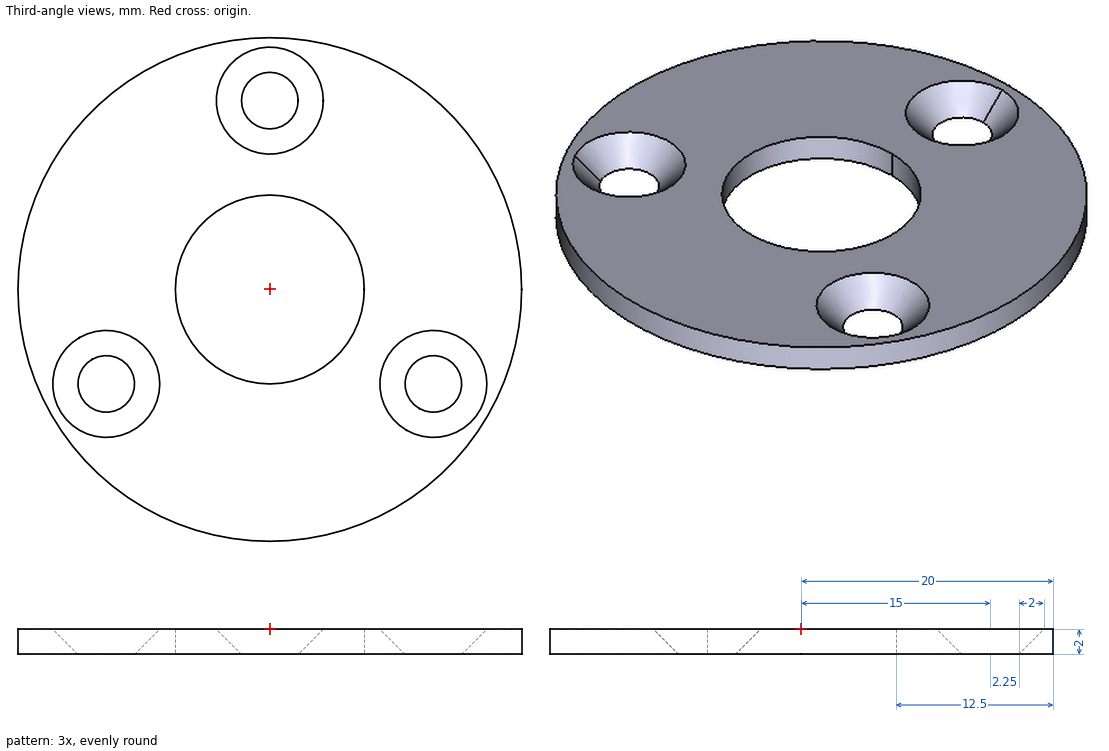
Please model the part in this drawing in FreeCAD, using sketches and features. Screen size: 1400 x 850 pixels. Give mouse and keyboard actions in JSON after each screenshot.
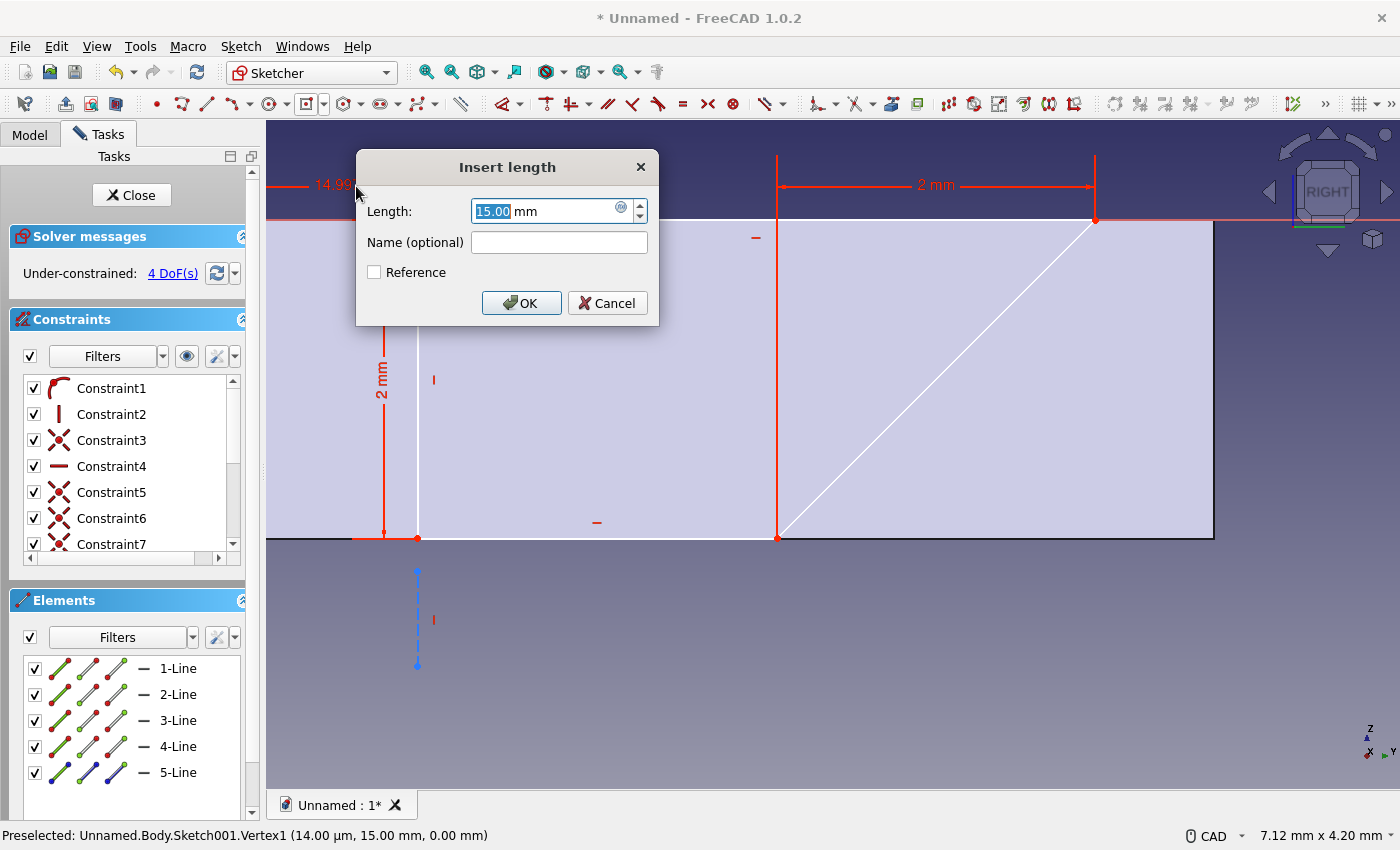
{"action": "type", "text": "15"}
{"action": "key", "text": "Return"}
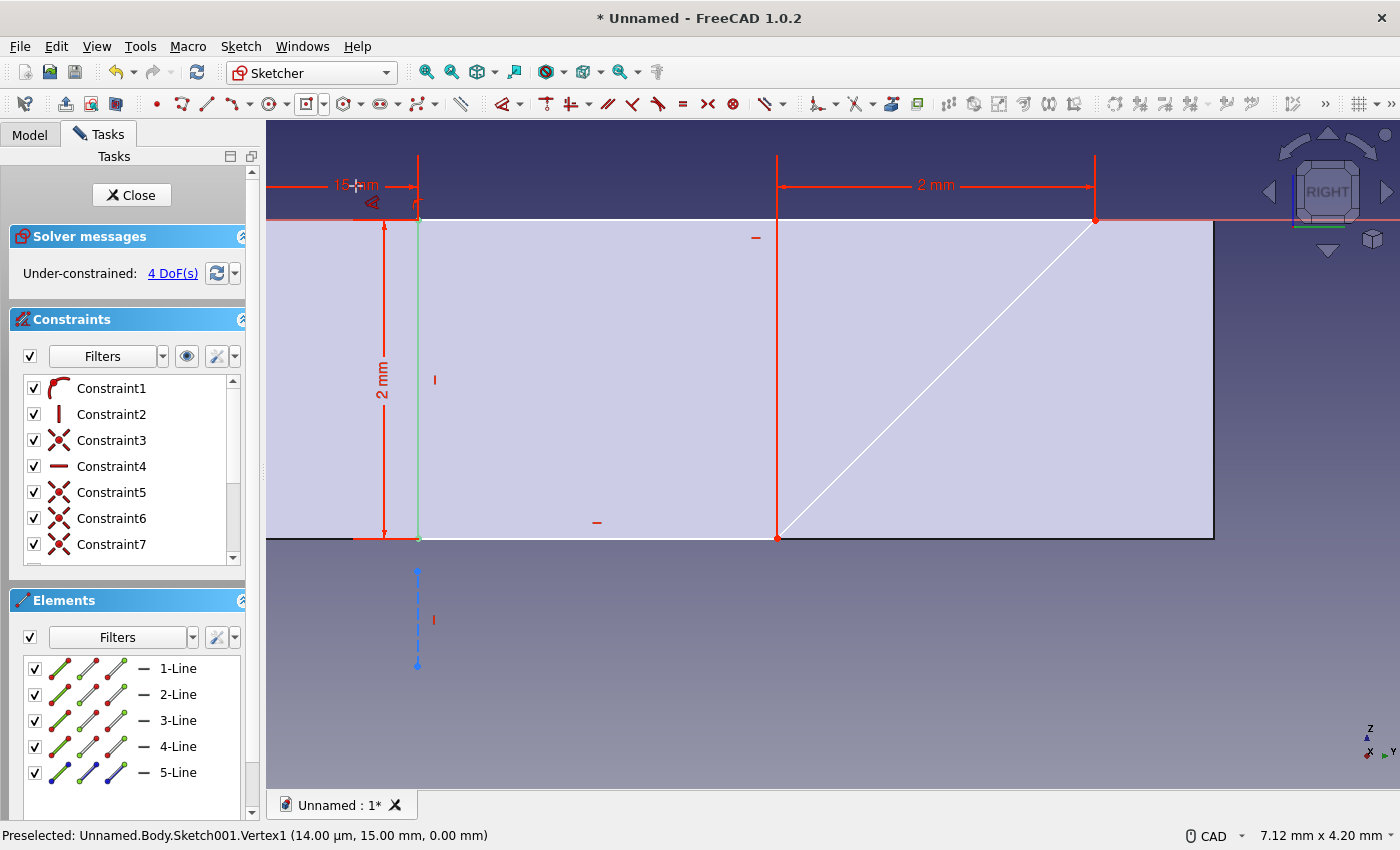
{"action": "left_click", "coordinate": [418, 572]}
{"action": "left_click", "coordinate": [356, 606]}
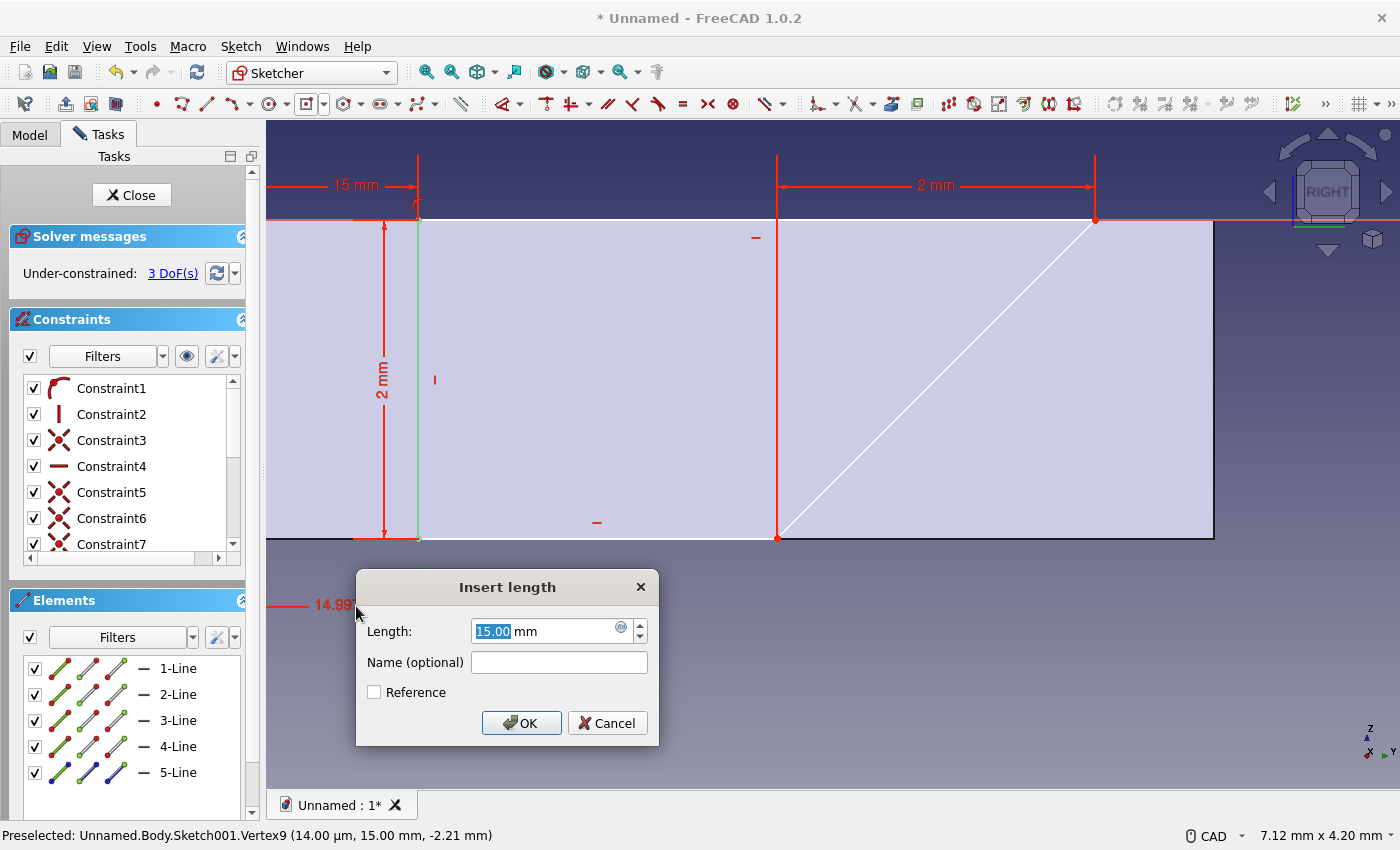
{"action": "type", "text": "15"}
{"action": "key", "text": "Return"}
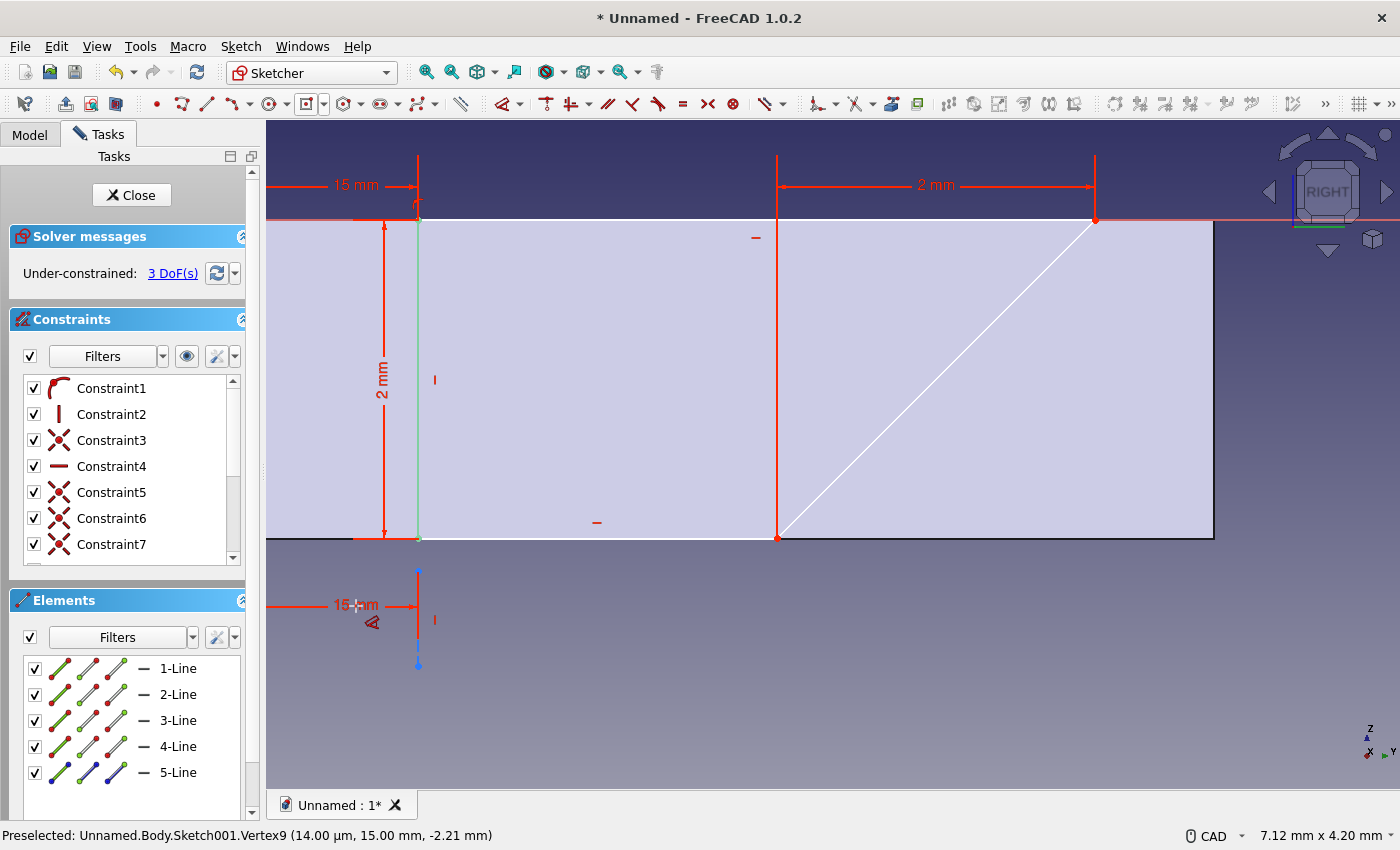
{"action": "left_click", "coordinate": [526, 539]}
{"action": "left_click", "coordinate": [598, 573]}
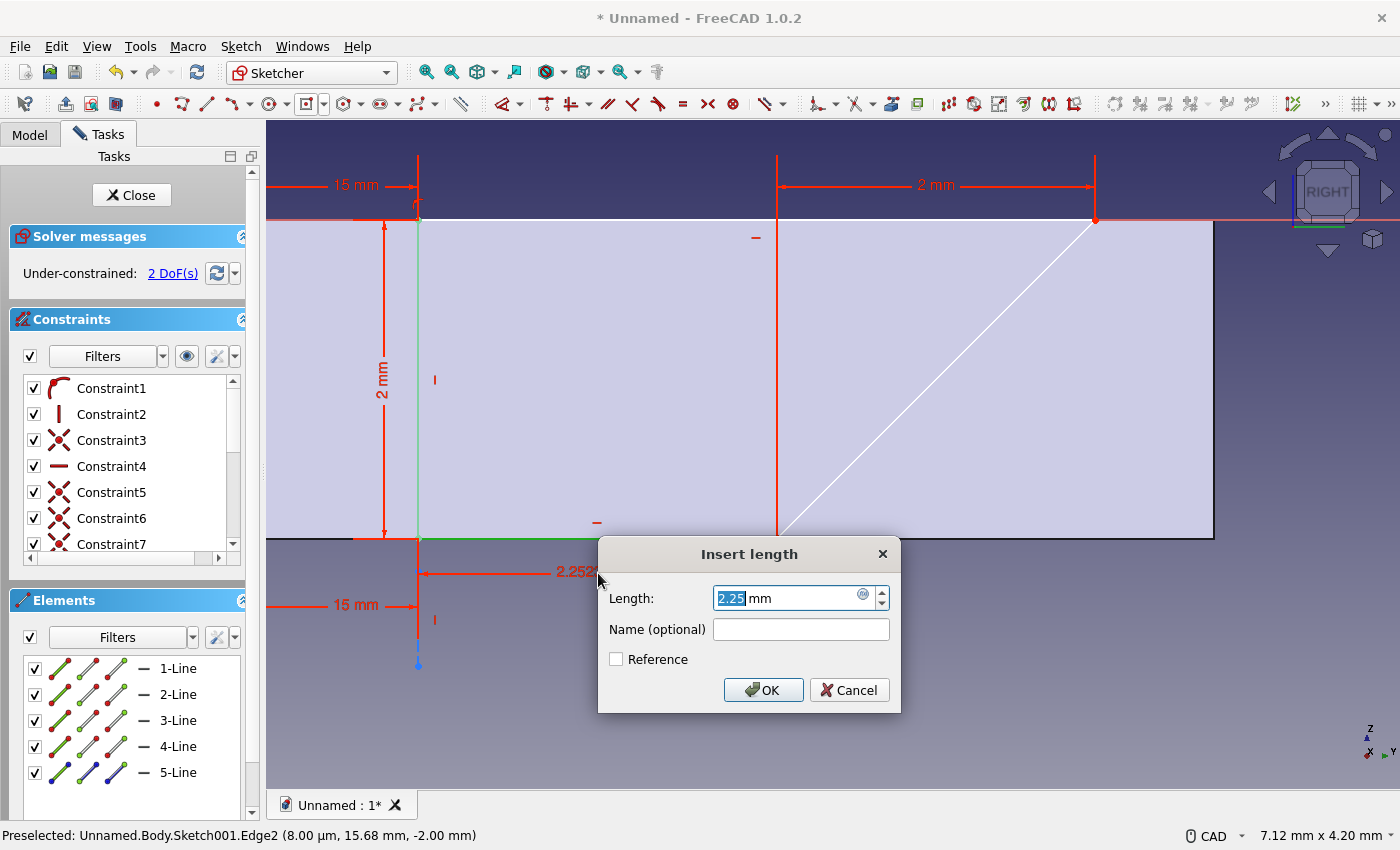
{"action": "type", "text": "2.25"}
{"action": "key", "text": "Return"}
{"action": "key", "text": "Escape"}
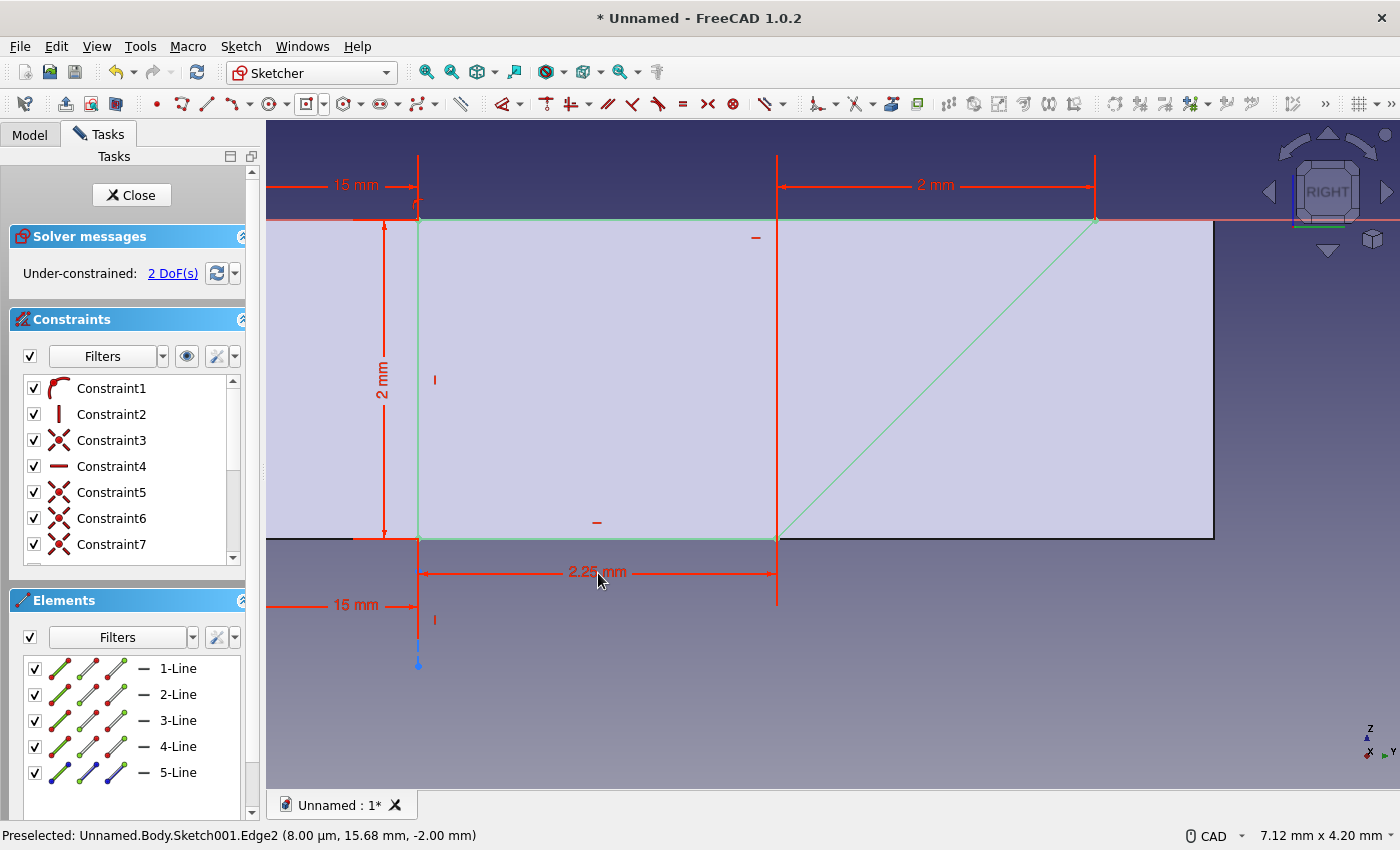
{"action": "left_click", "coordinate": [132, 195]}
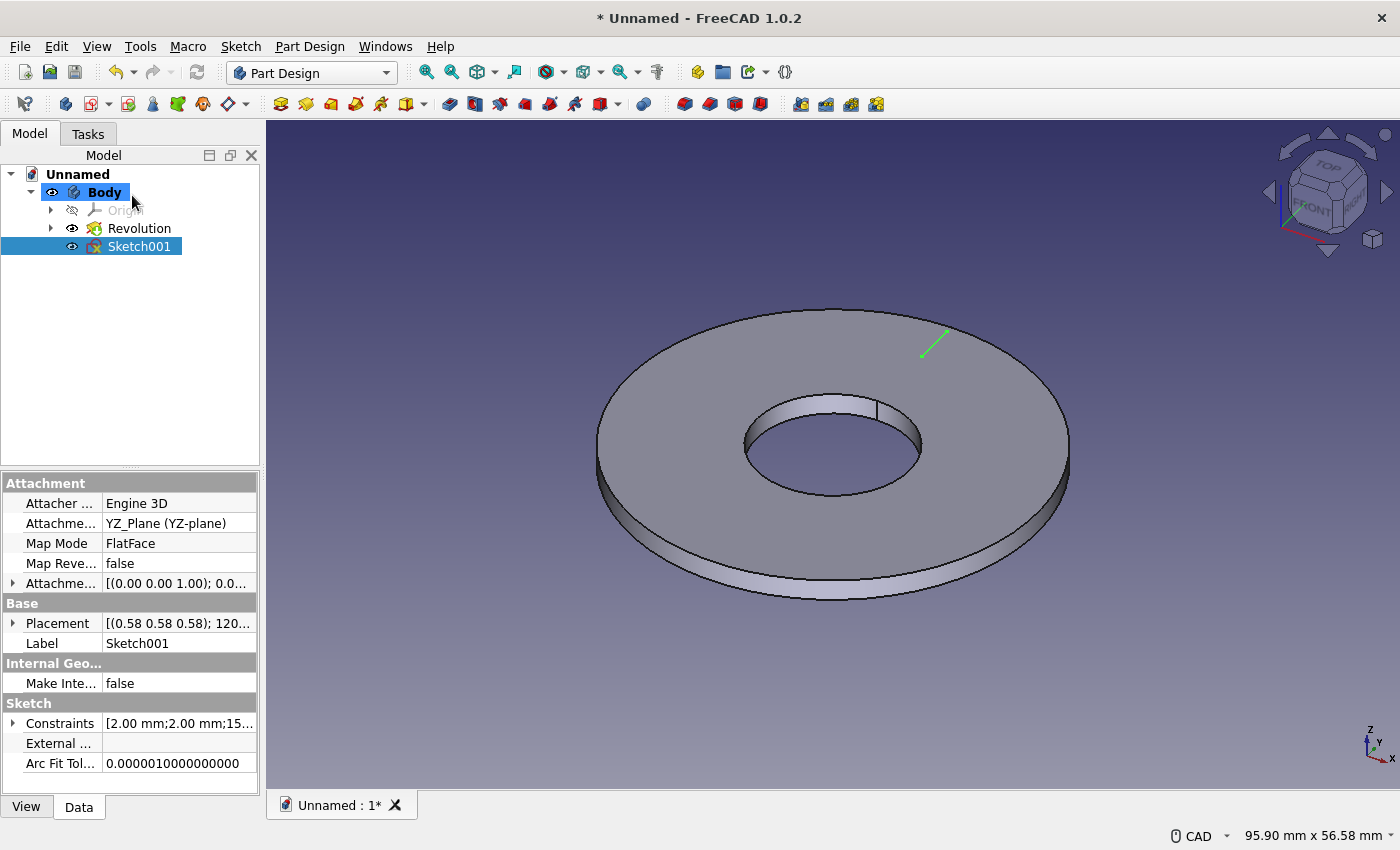
{"action": "left_click", "coordinate": [500, 104]}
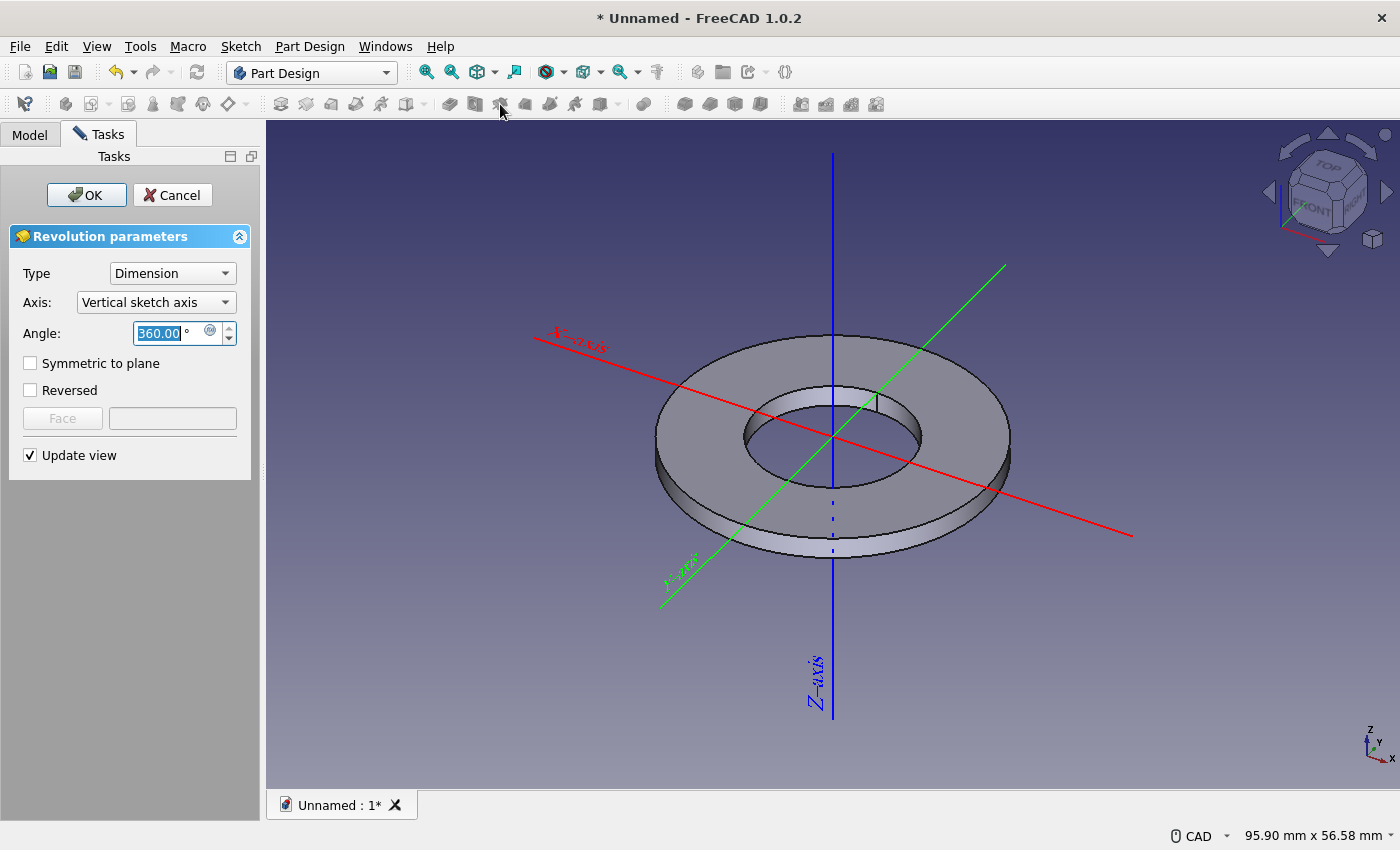
{"action": "left_click", "coordinate": [157, 302]}